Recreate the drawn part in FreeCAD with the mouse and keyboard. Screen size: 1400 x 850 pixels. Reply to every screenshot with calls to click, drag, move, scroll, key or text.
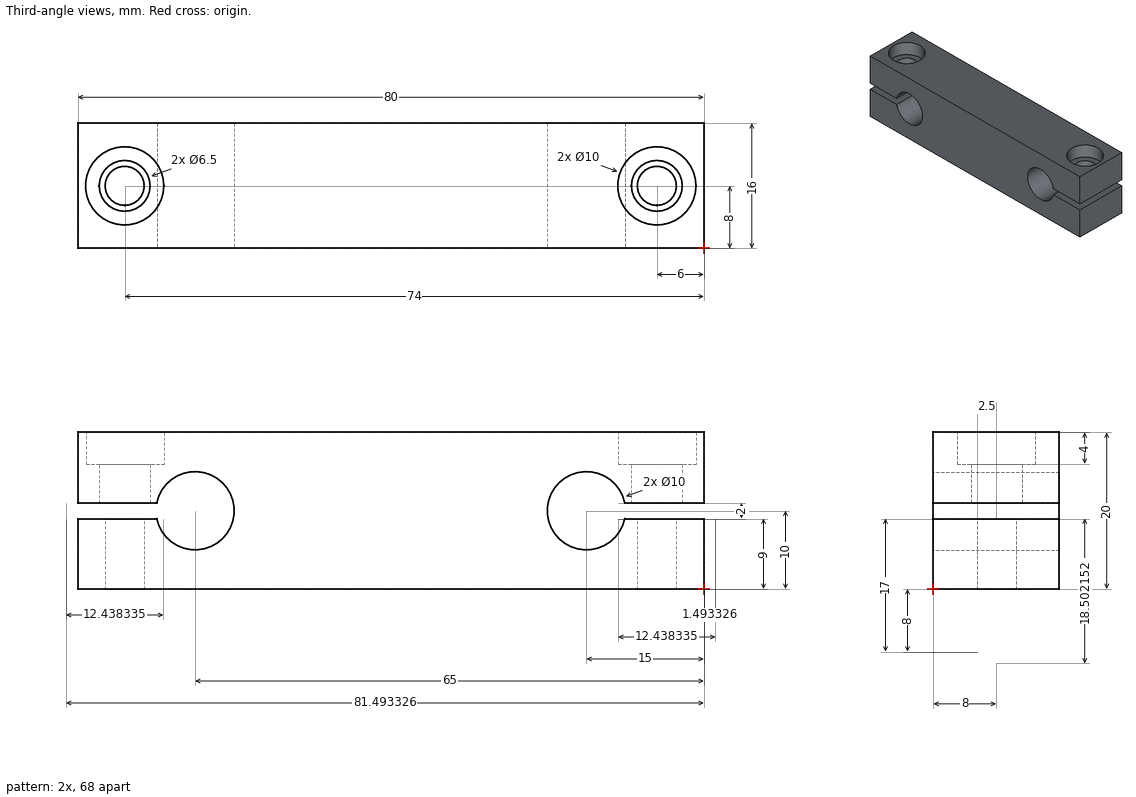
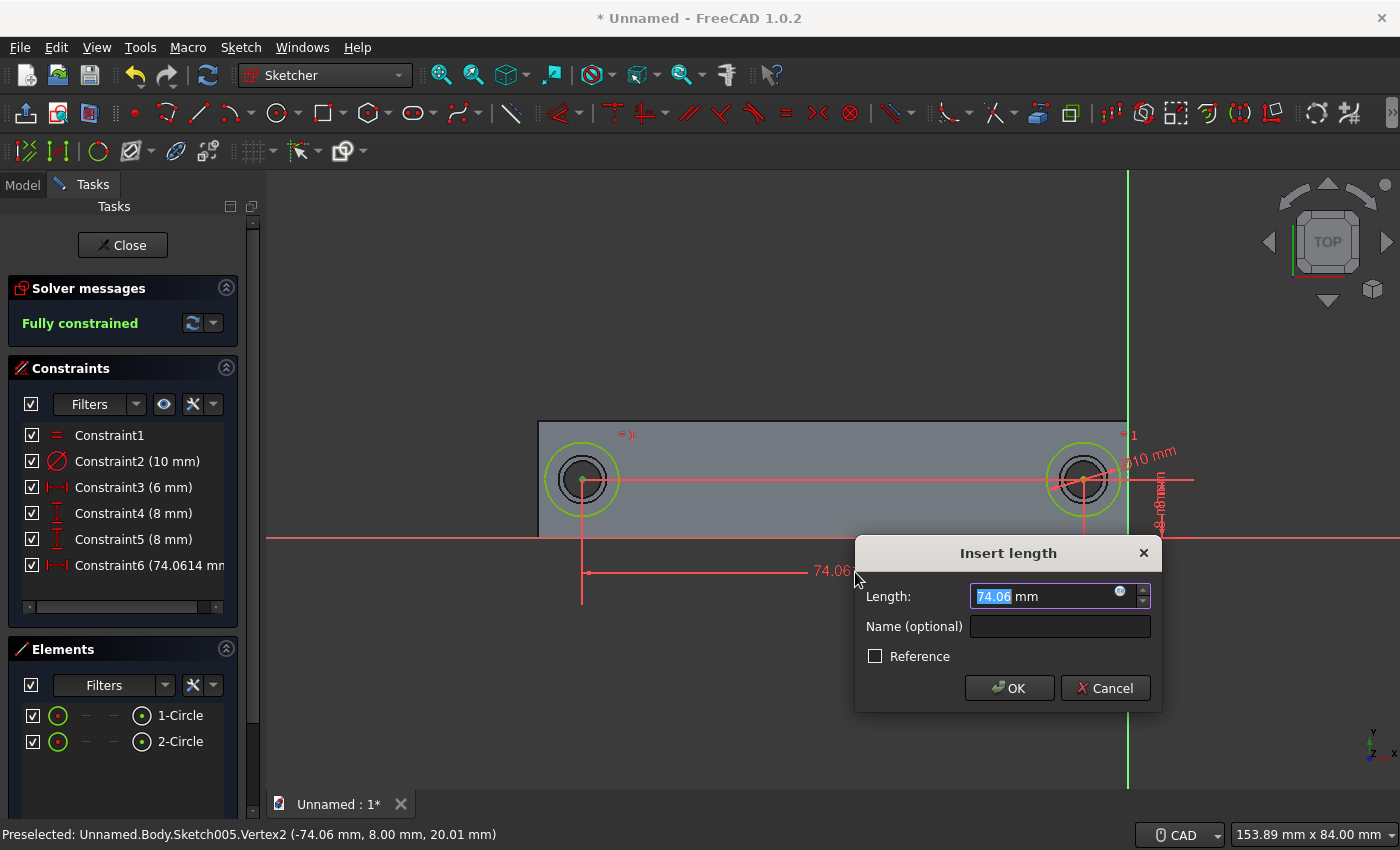
text(74)
key(Return)
key(Escape)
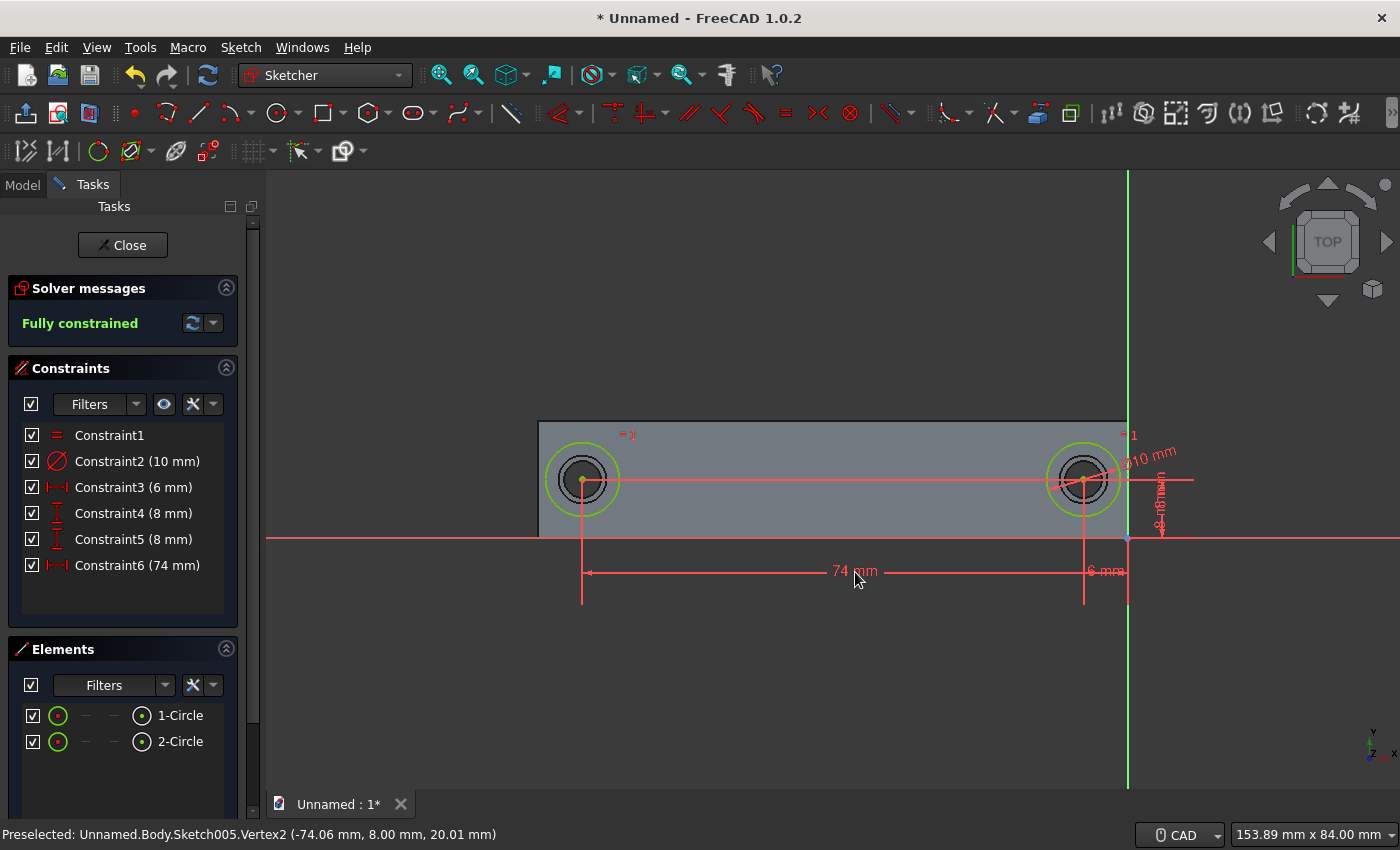
click(123, 245)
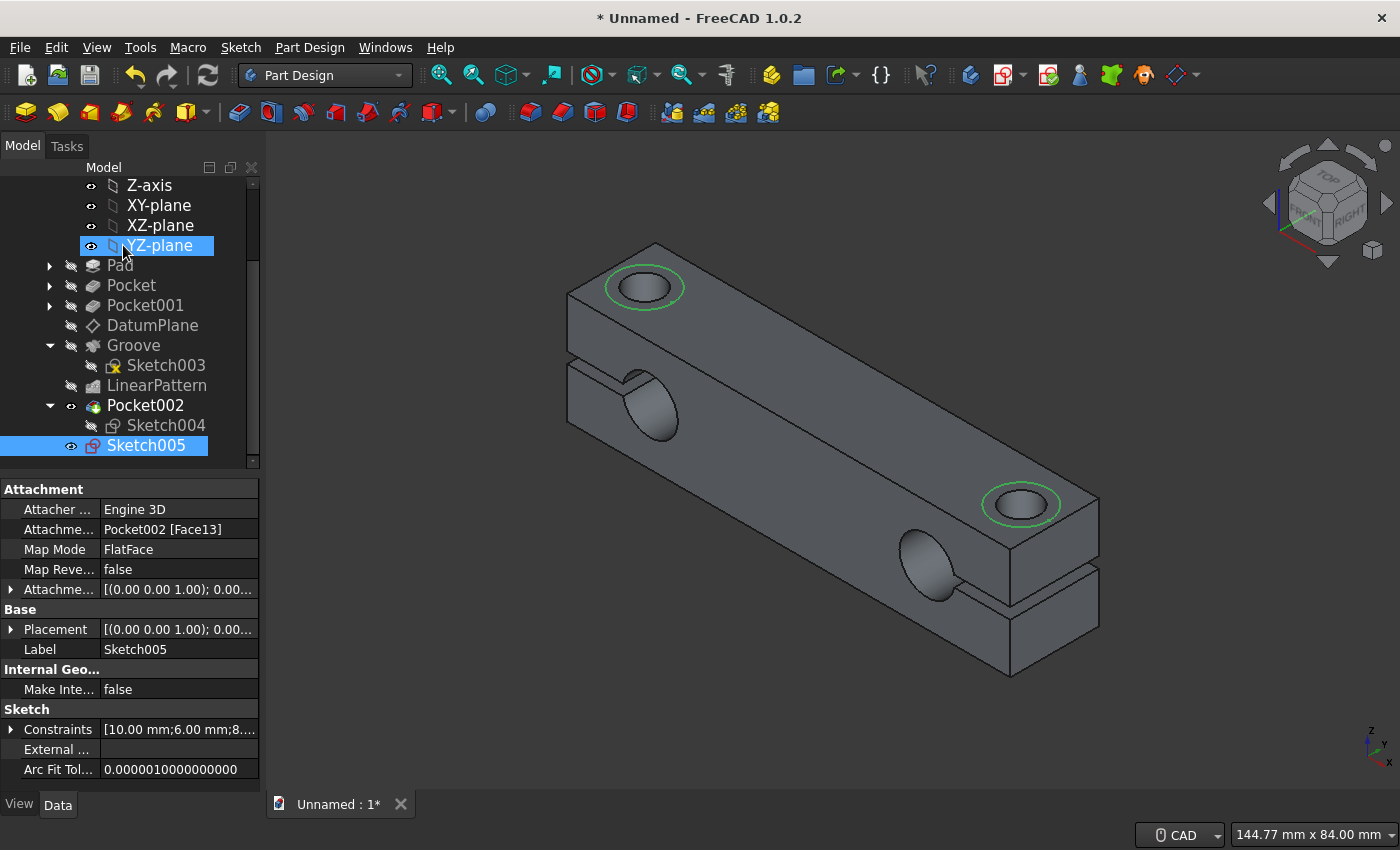
click(240, 112)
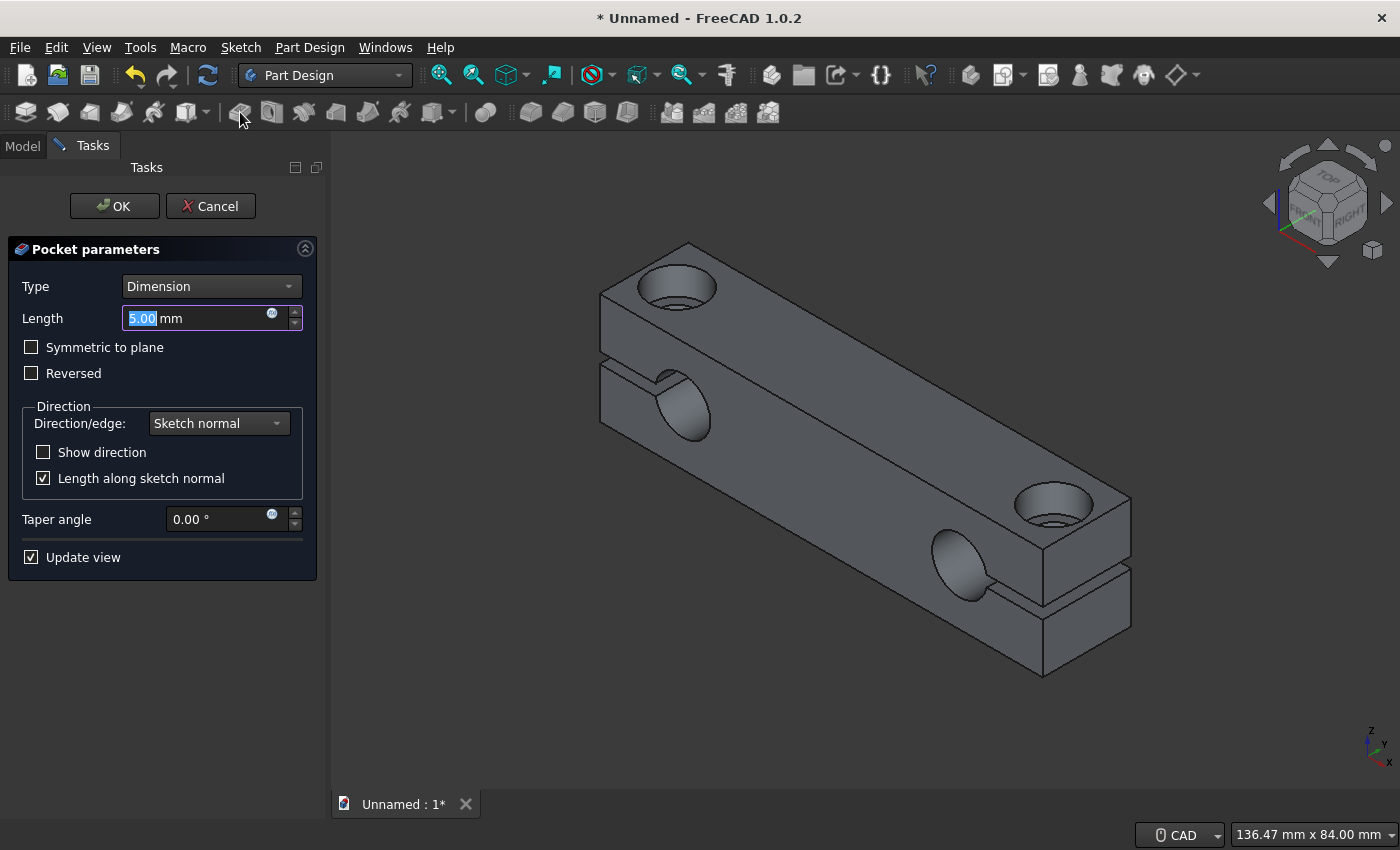
text(4)
key(Tab)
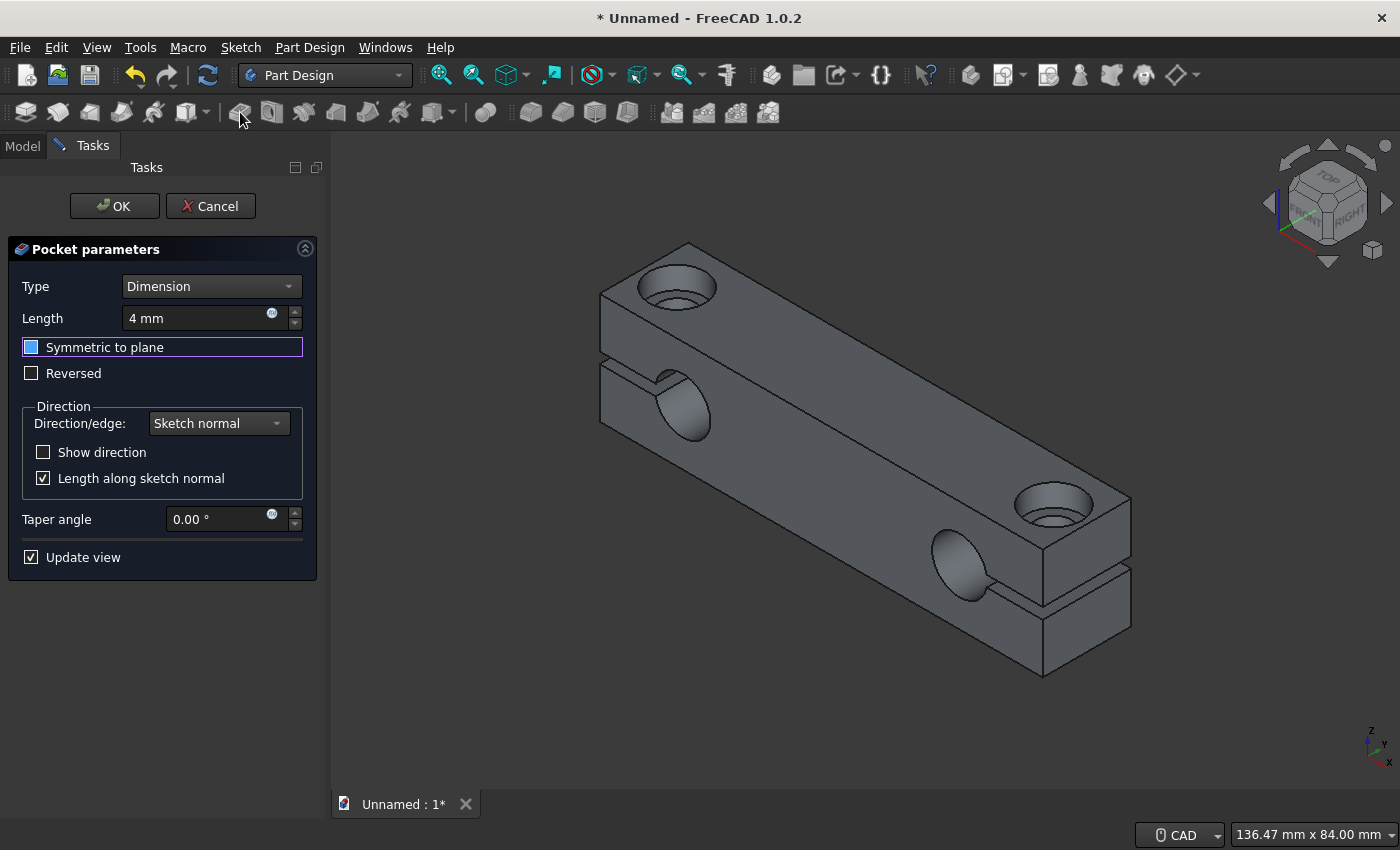
click(115, 206)